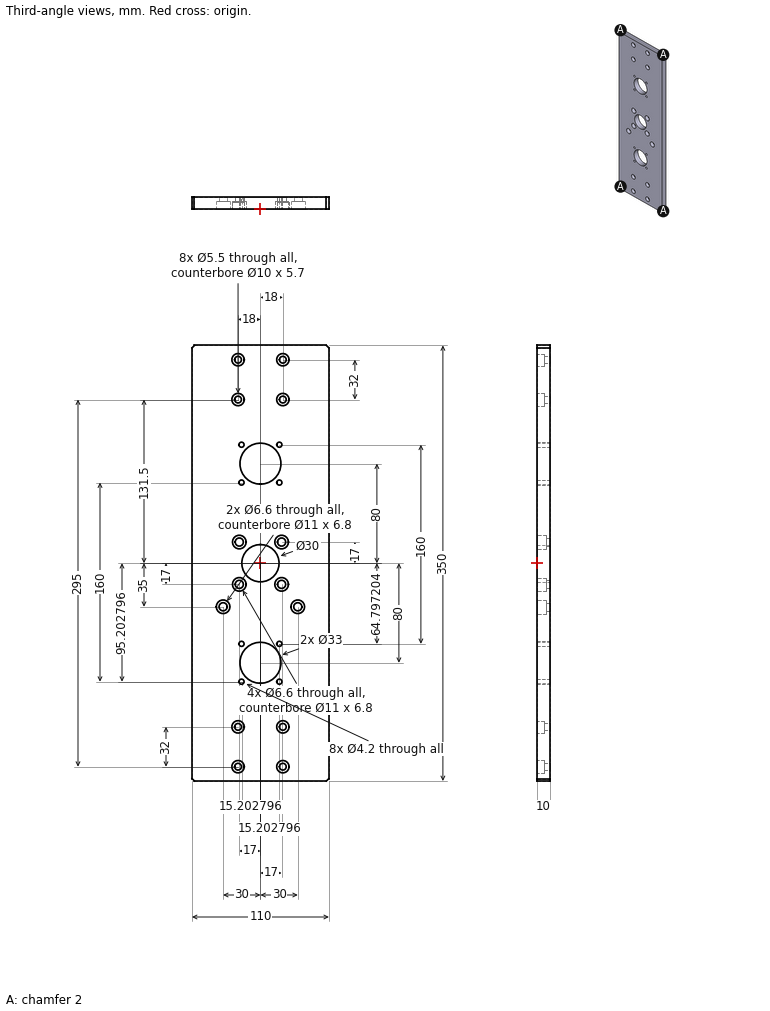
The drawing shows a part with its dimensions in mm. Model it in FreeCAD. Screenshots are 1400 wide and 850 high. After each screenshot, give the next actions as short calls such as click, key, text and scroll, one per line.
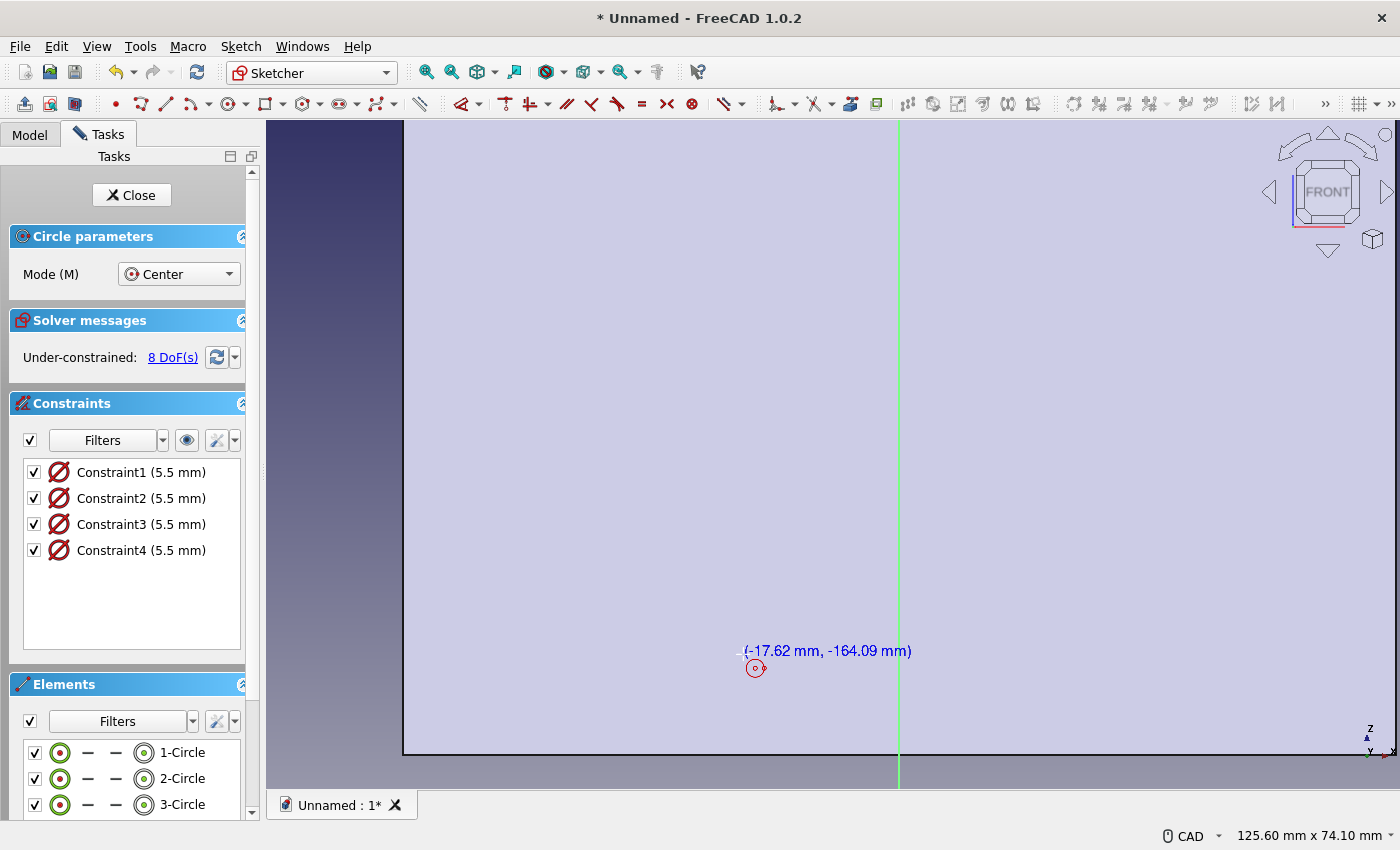
scroll(743, 655, down, 10)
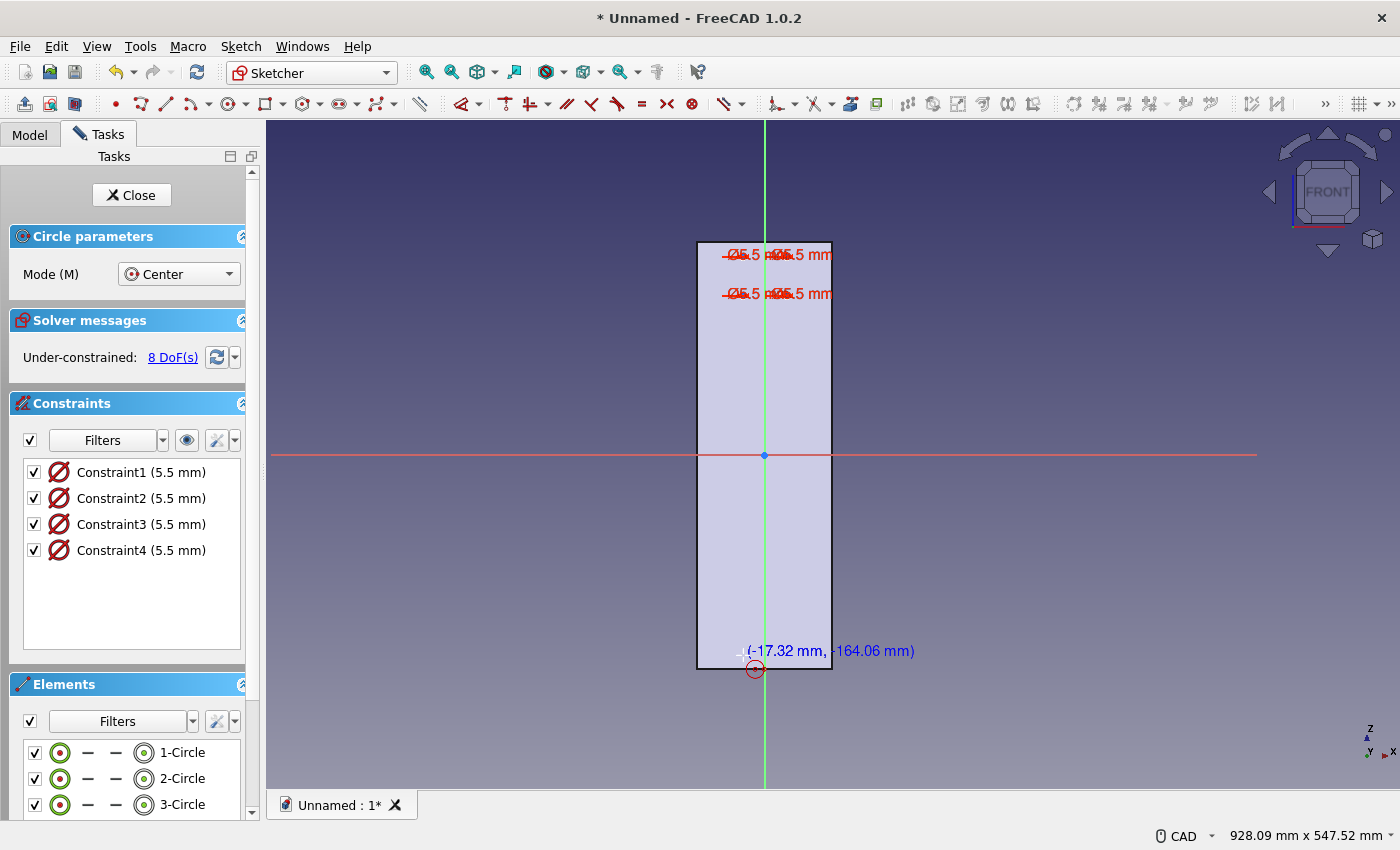
click(743, 655)
move(745, 653)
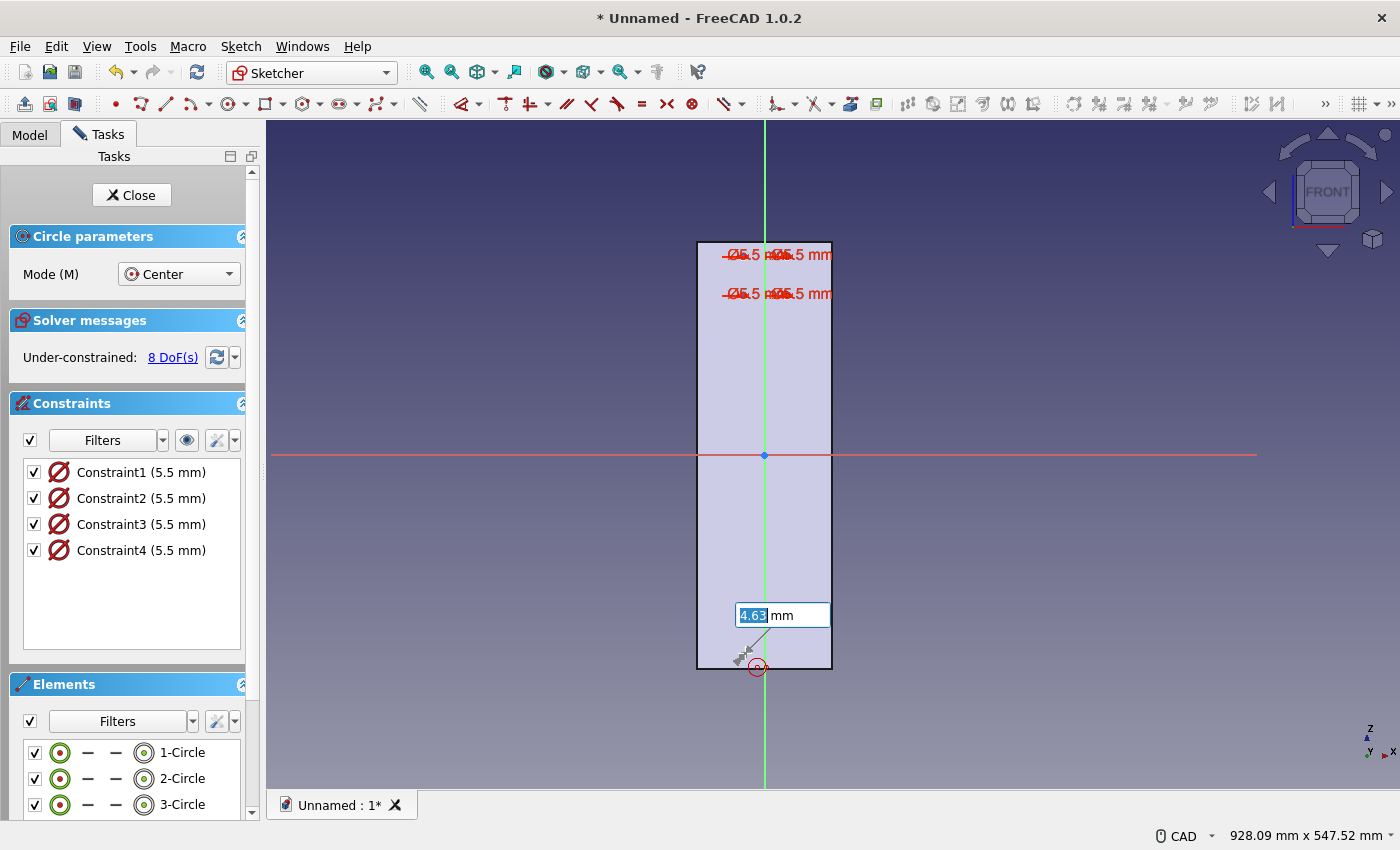
text(5.5)
key(Return)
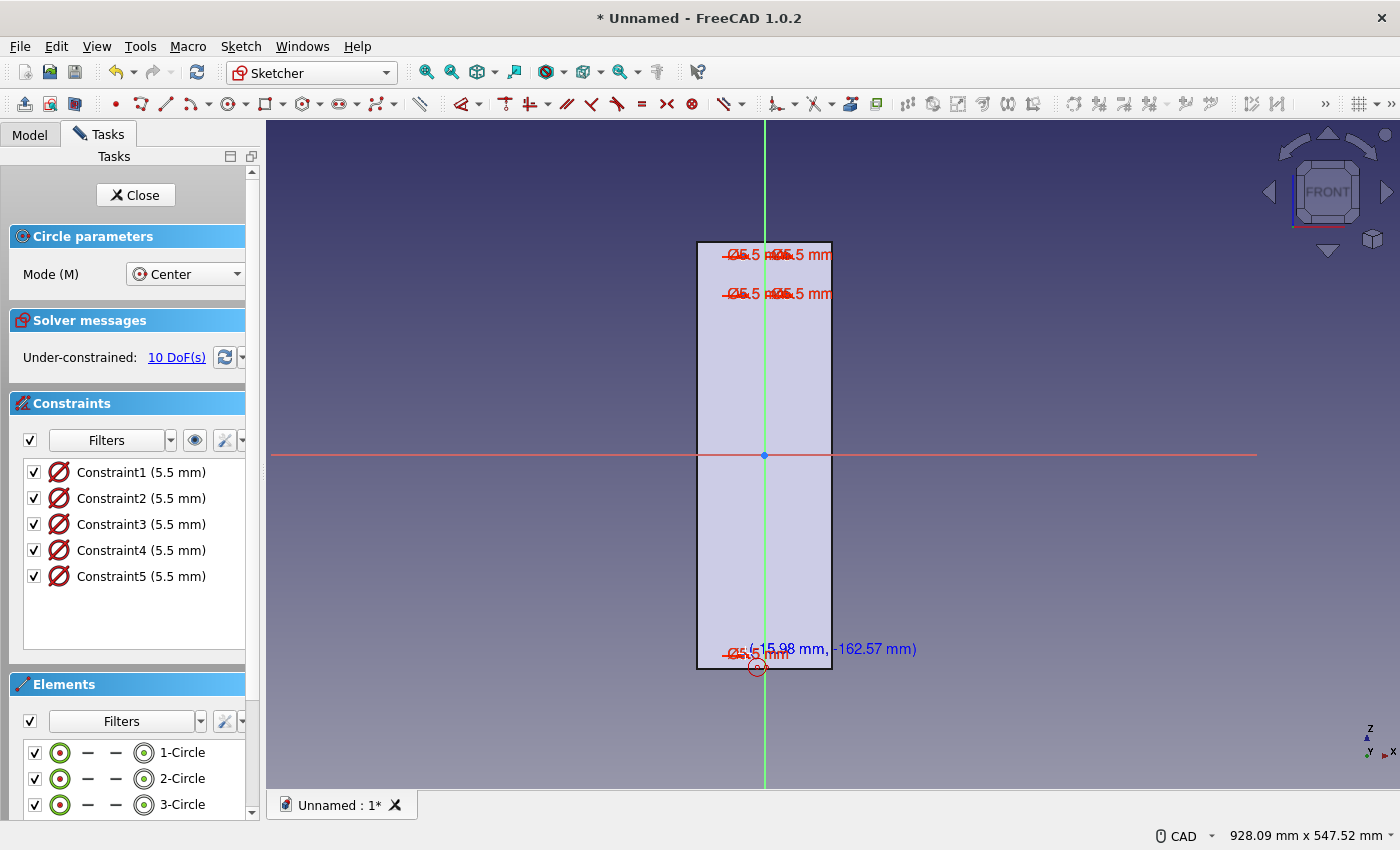
scroll(743, 616, up, 10)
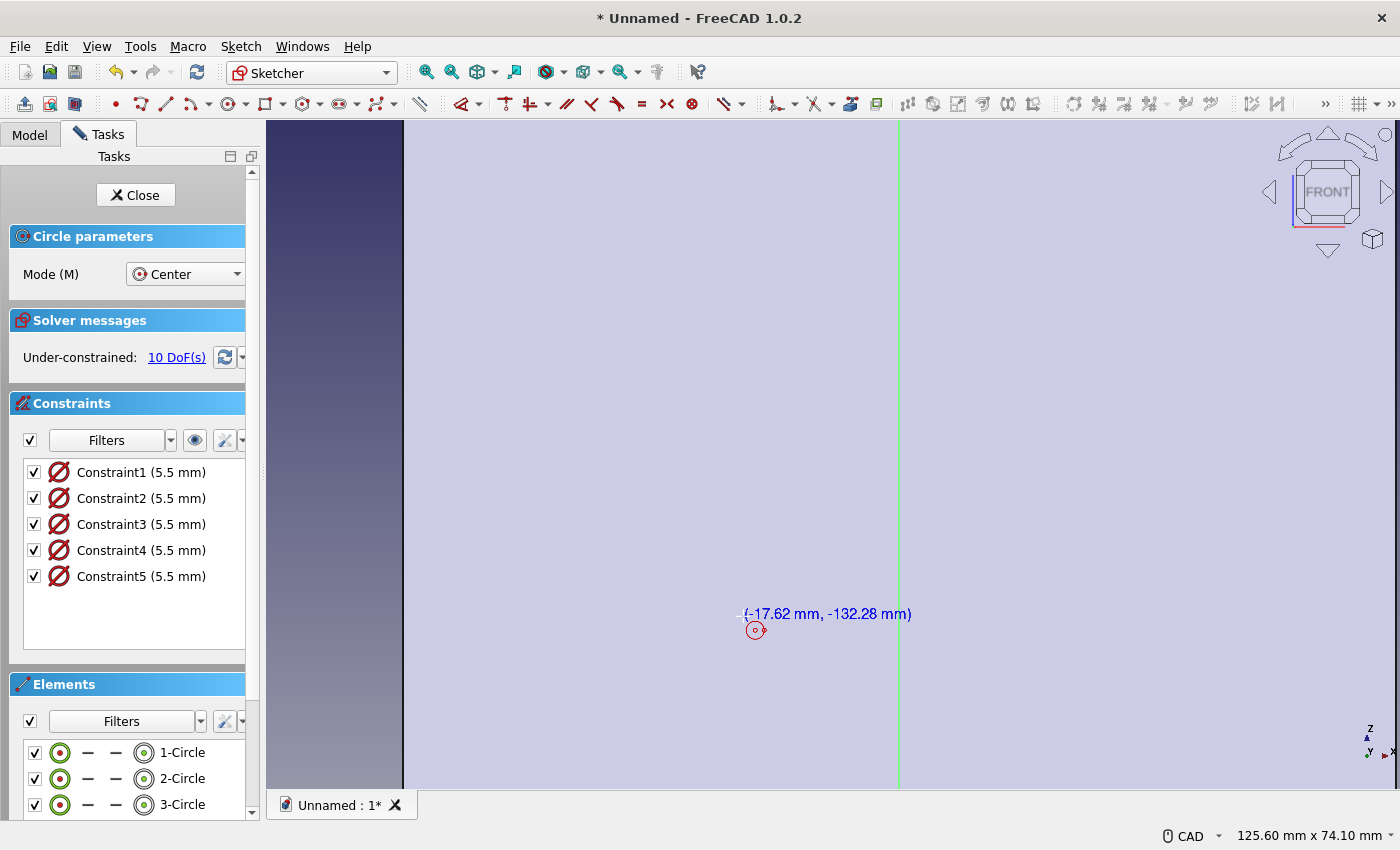
scroll(743, 616, down, 10)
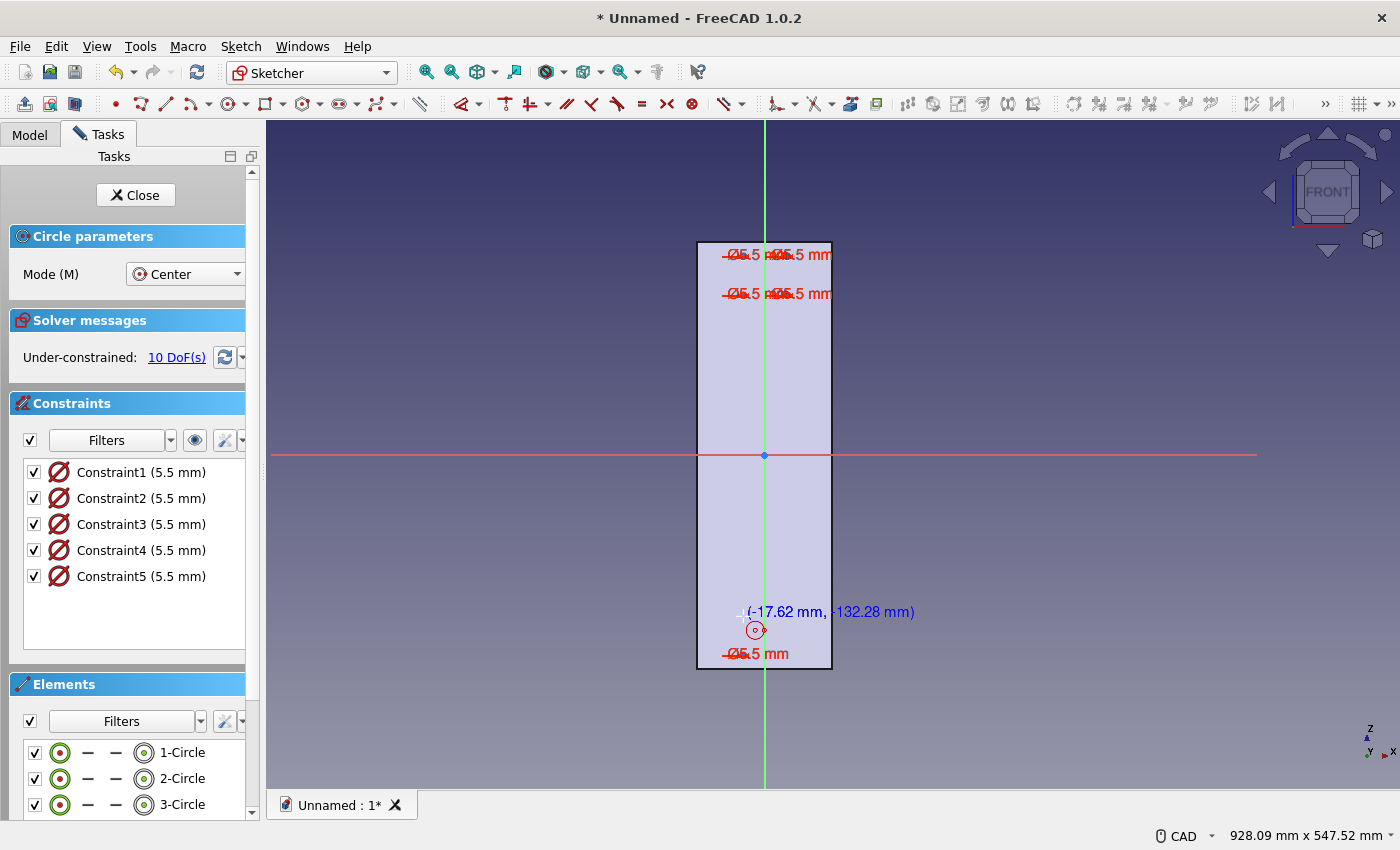
click(743, 616)
move(745, 614)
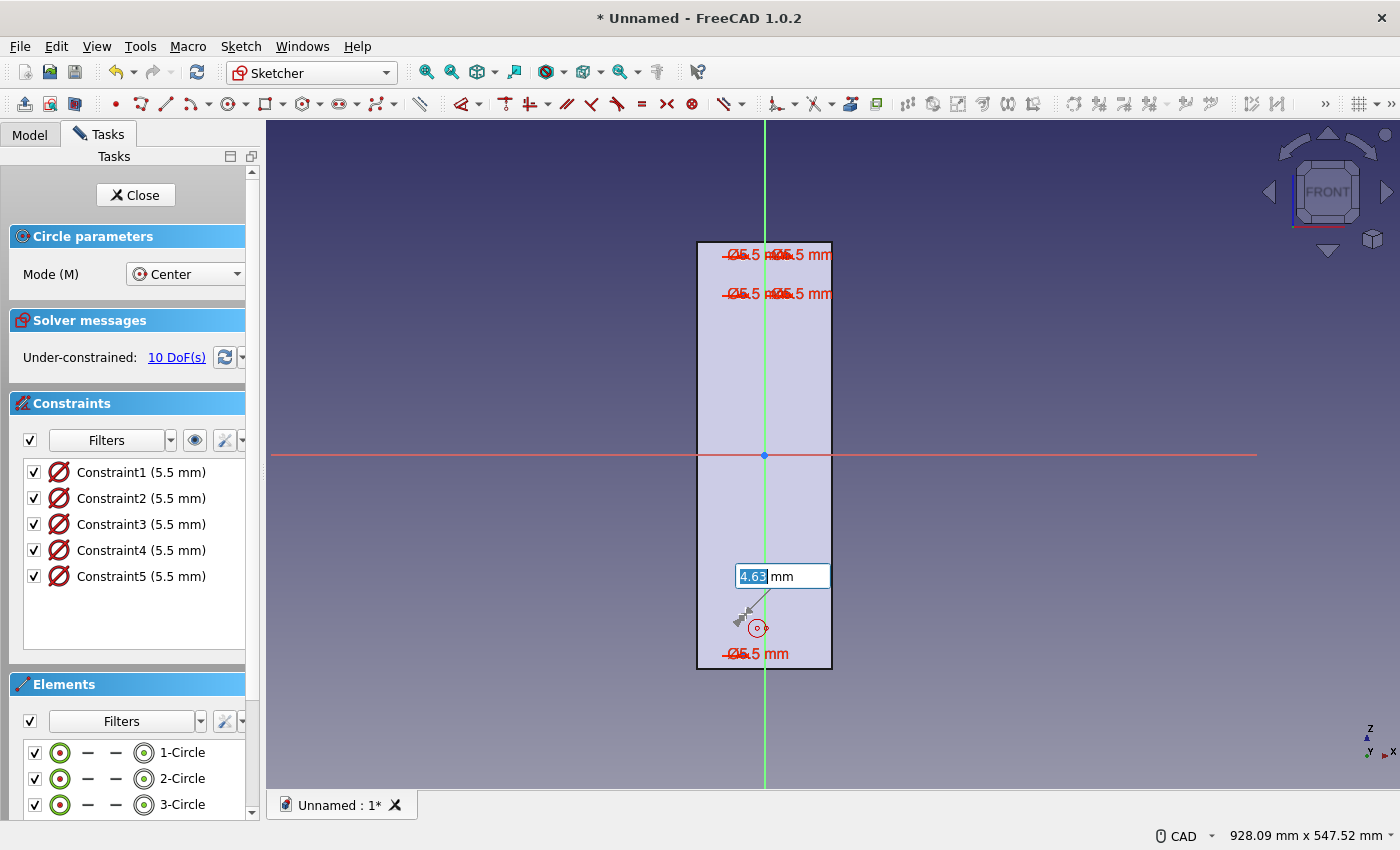
text(5.5)
key(Return)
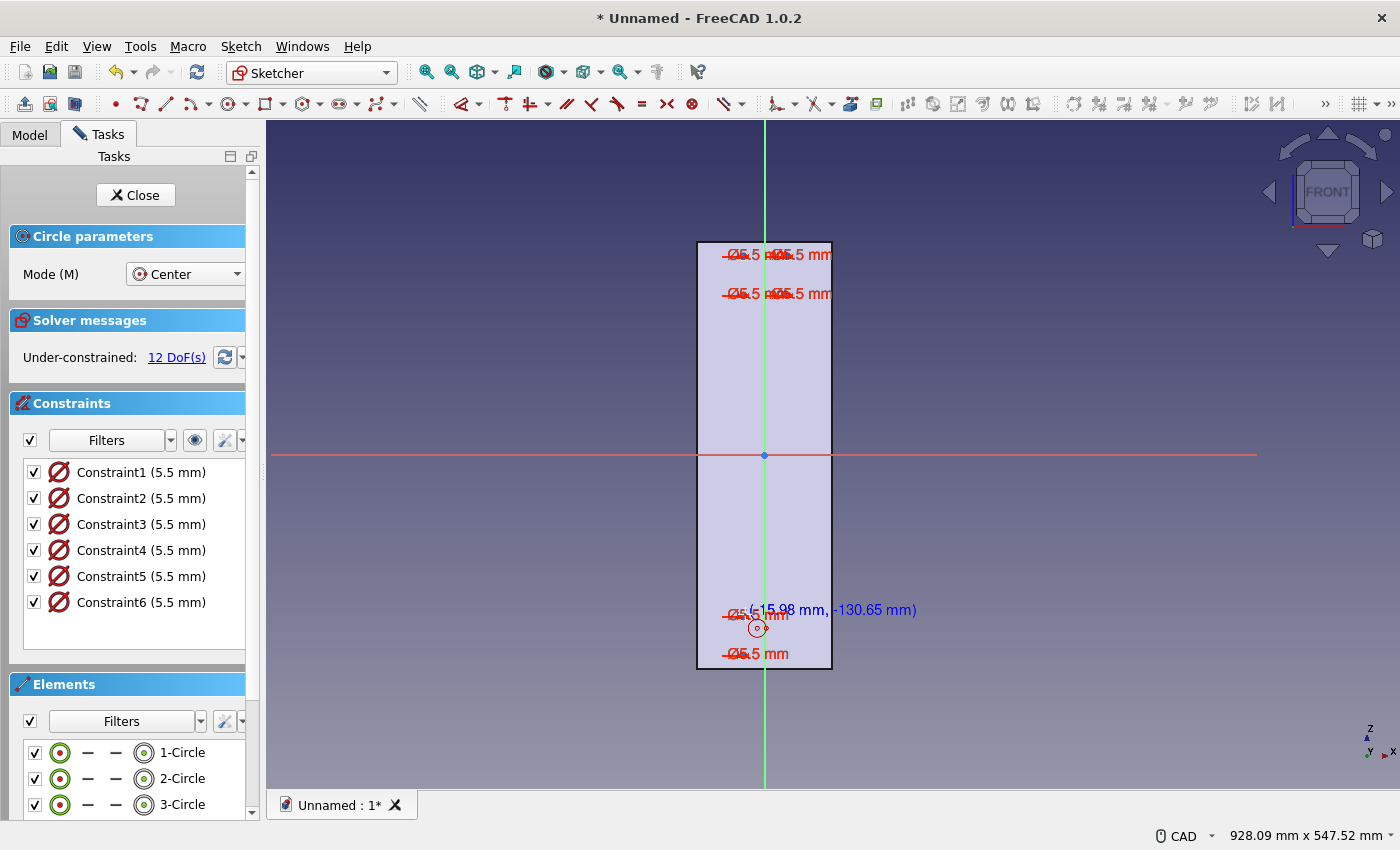
scroll(787, 655, up, 10)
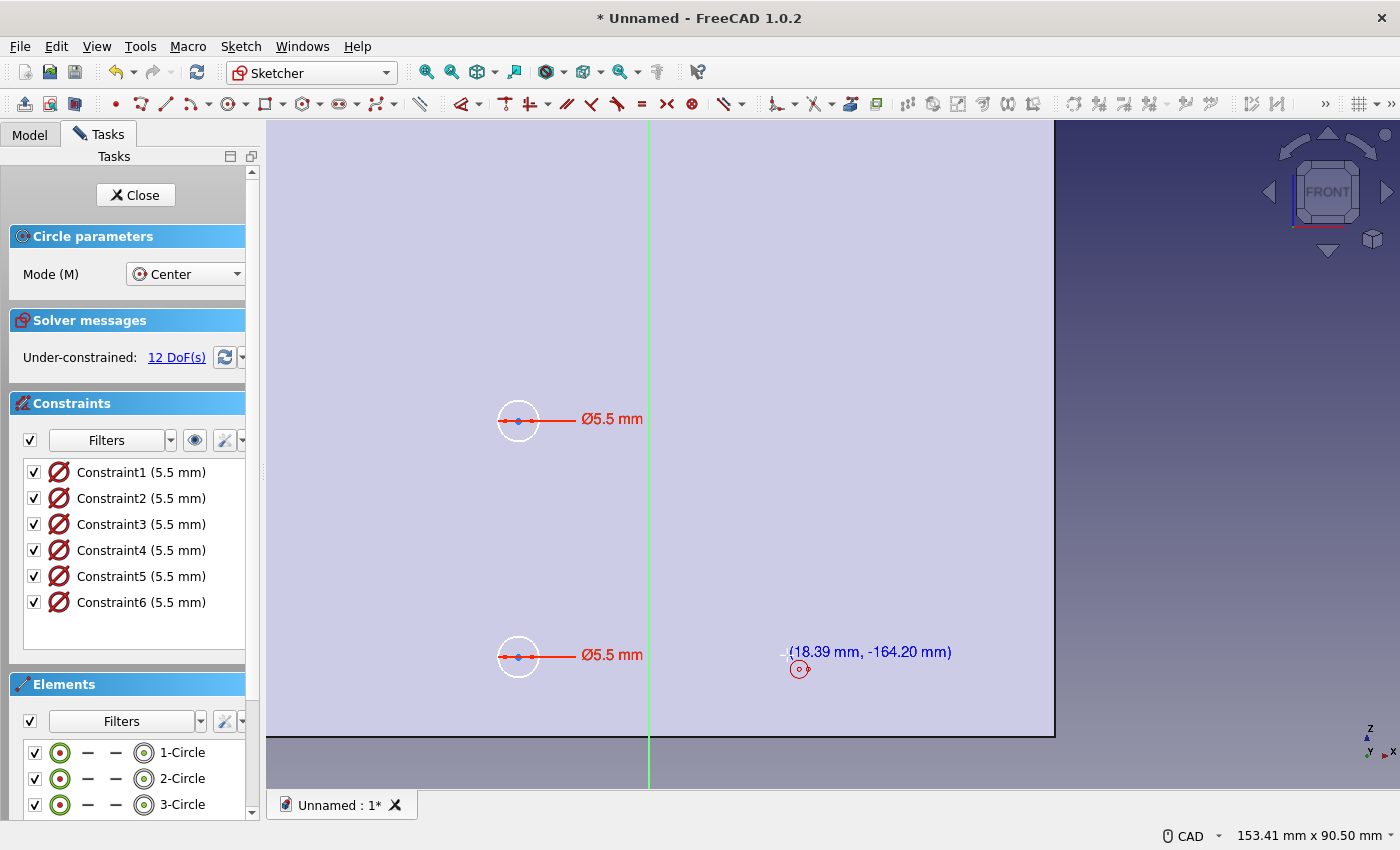
scroll(787, 655, down, 10)